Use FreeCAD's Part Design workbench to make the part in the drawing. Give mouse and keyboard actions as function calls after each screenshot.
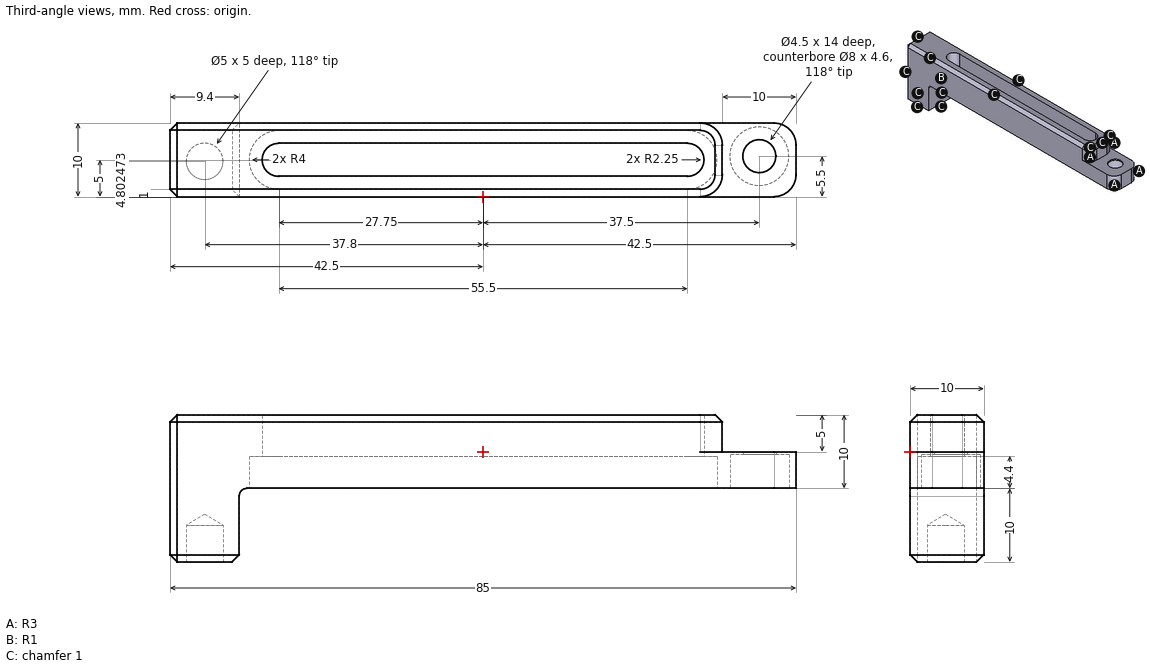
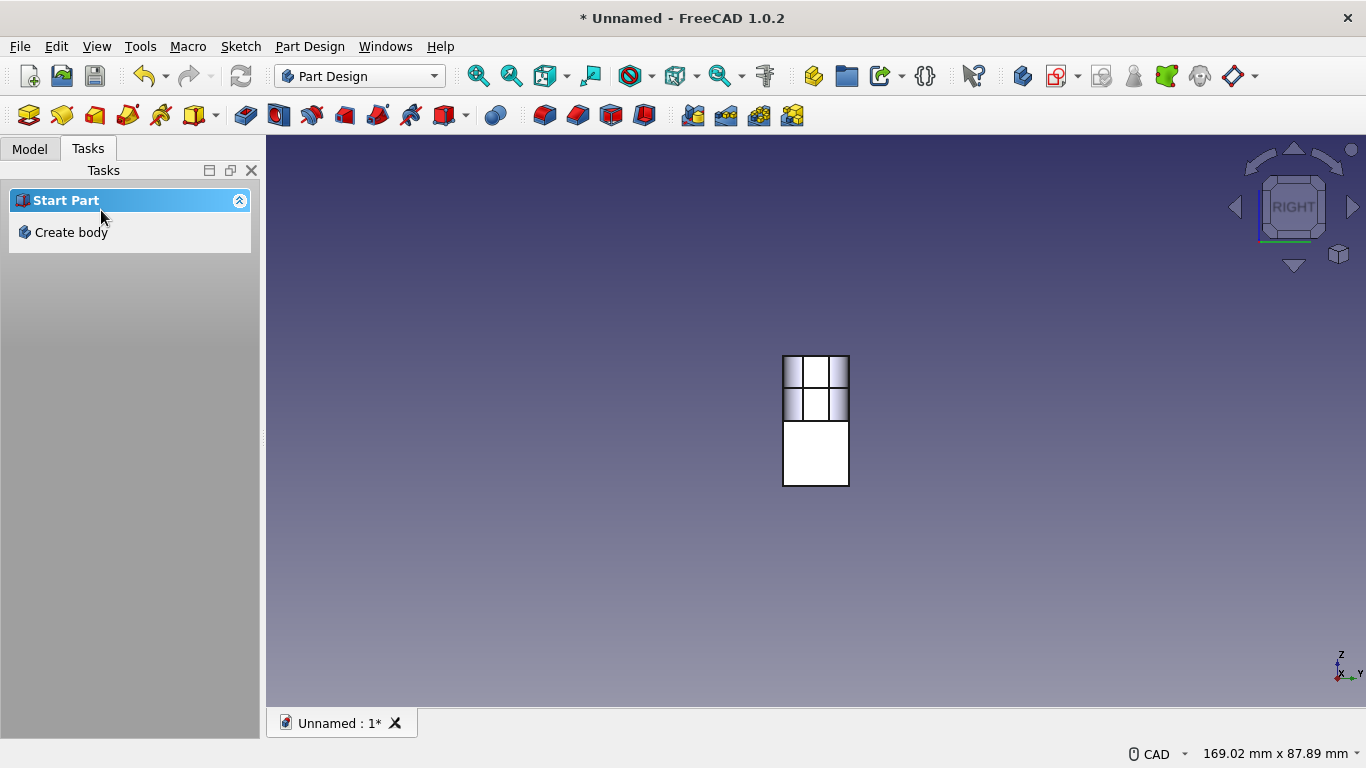
key(5)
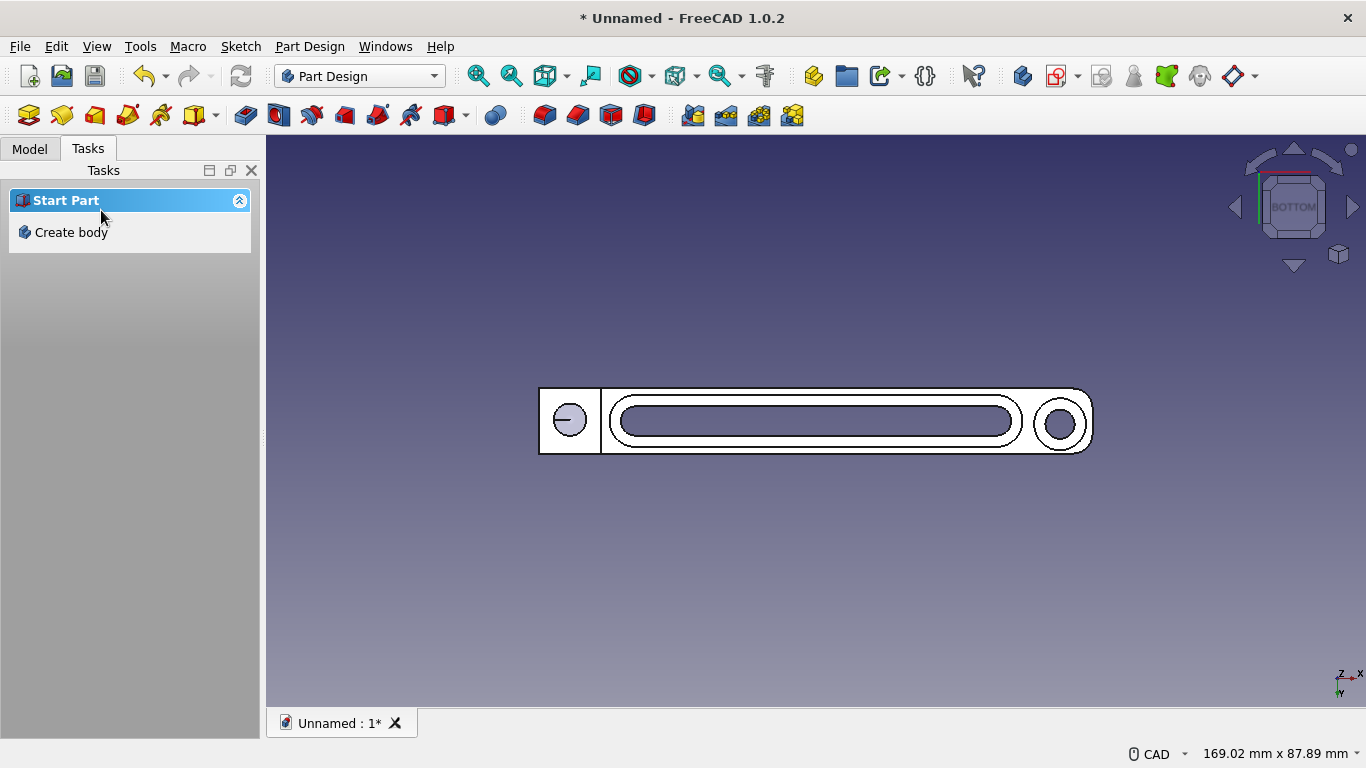
key(4)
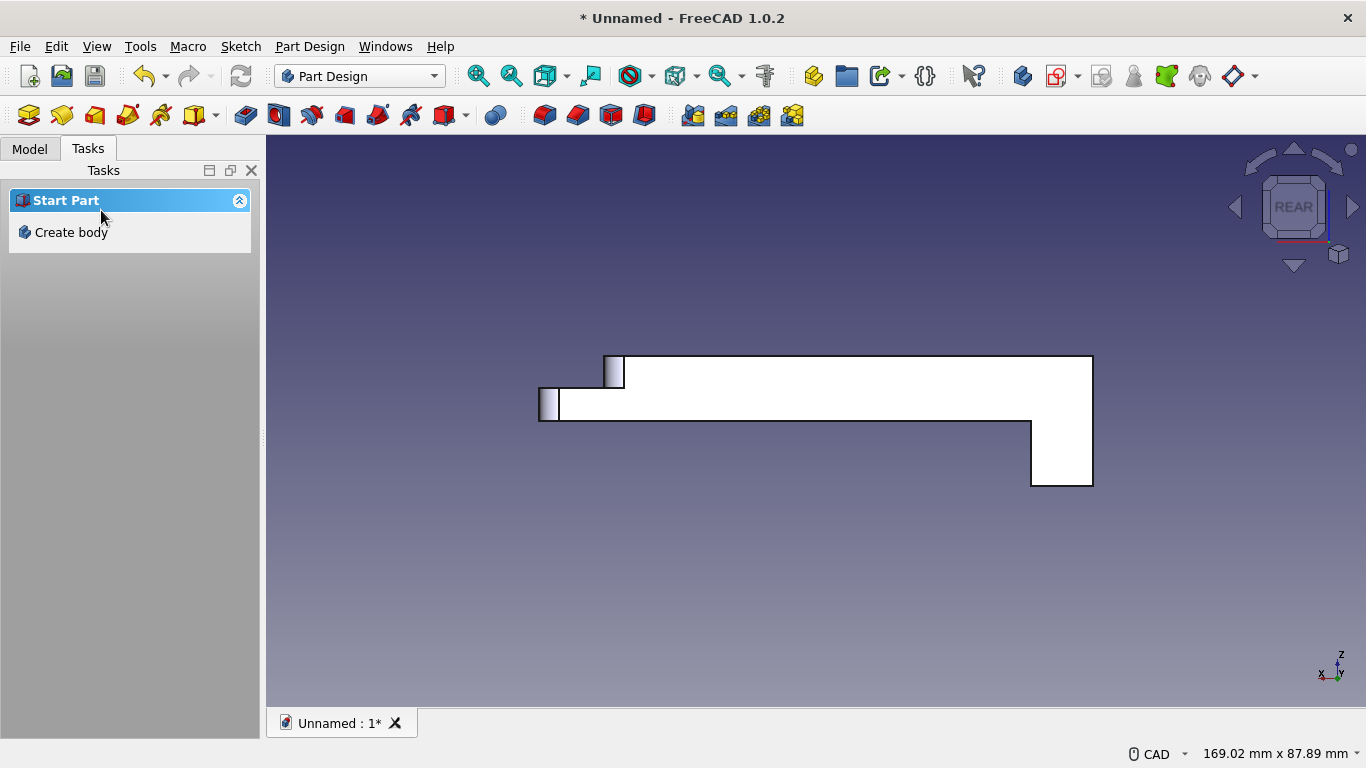
key(6)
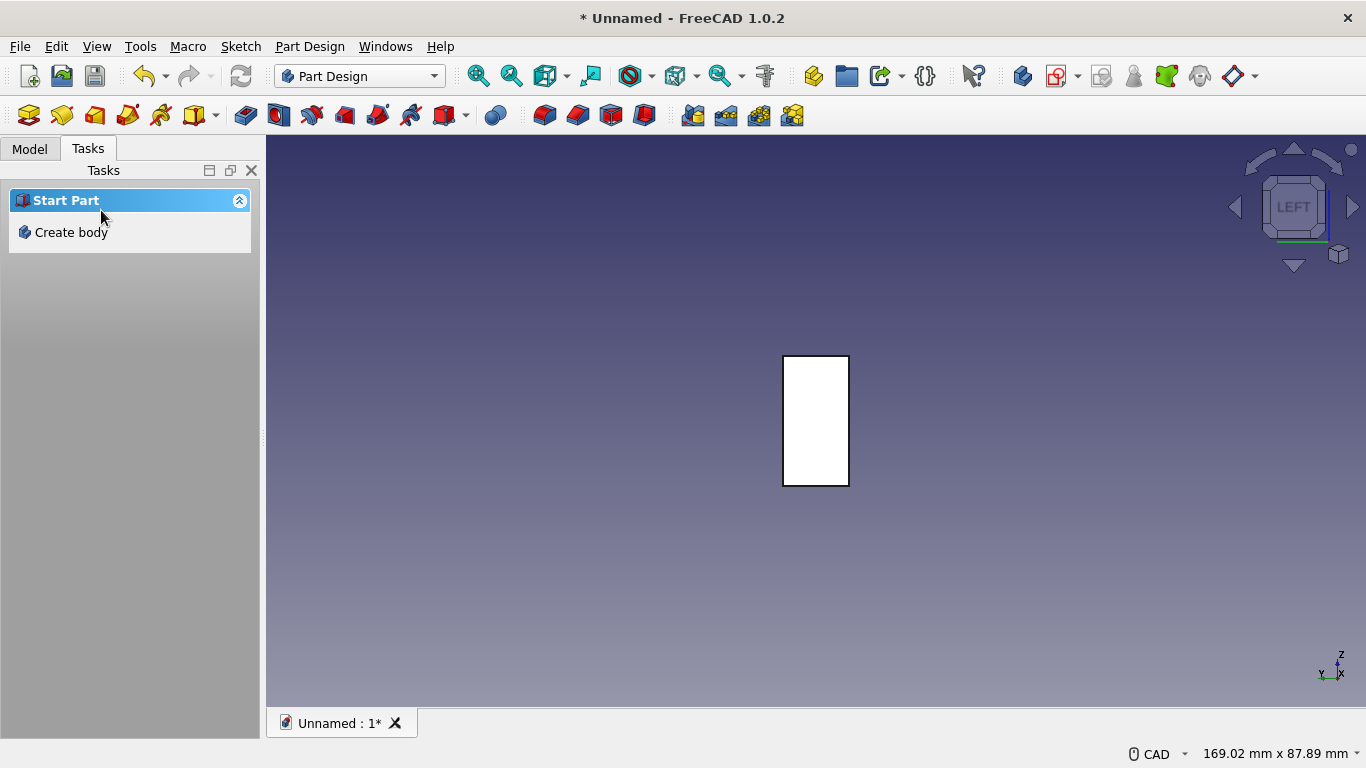
click(479, 76)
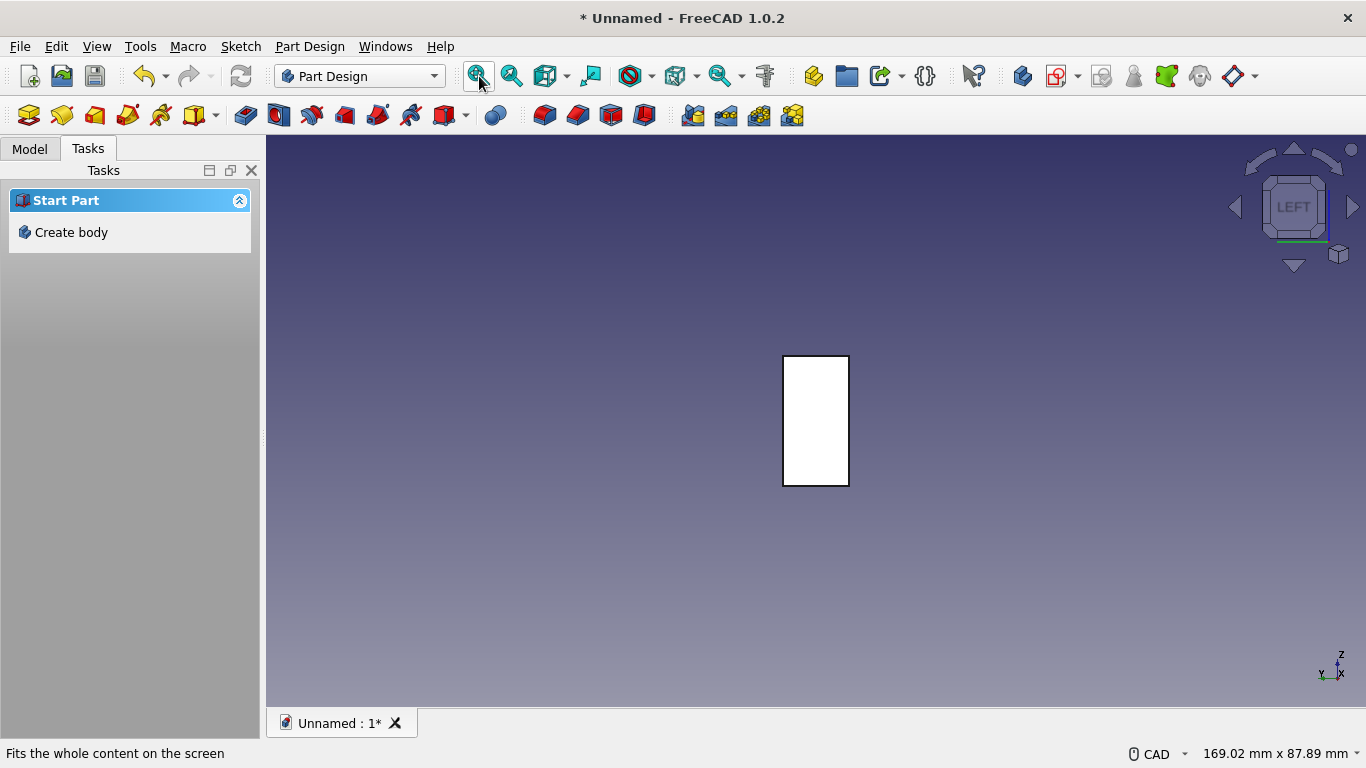
key(v)
key(3)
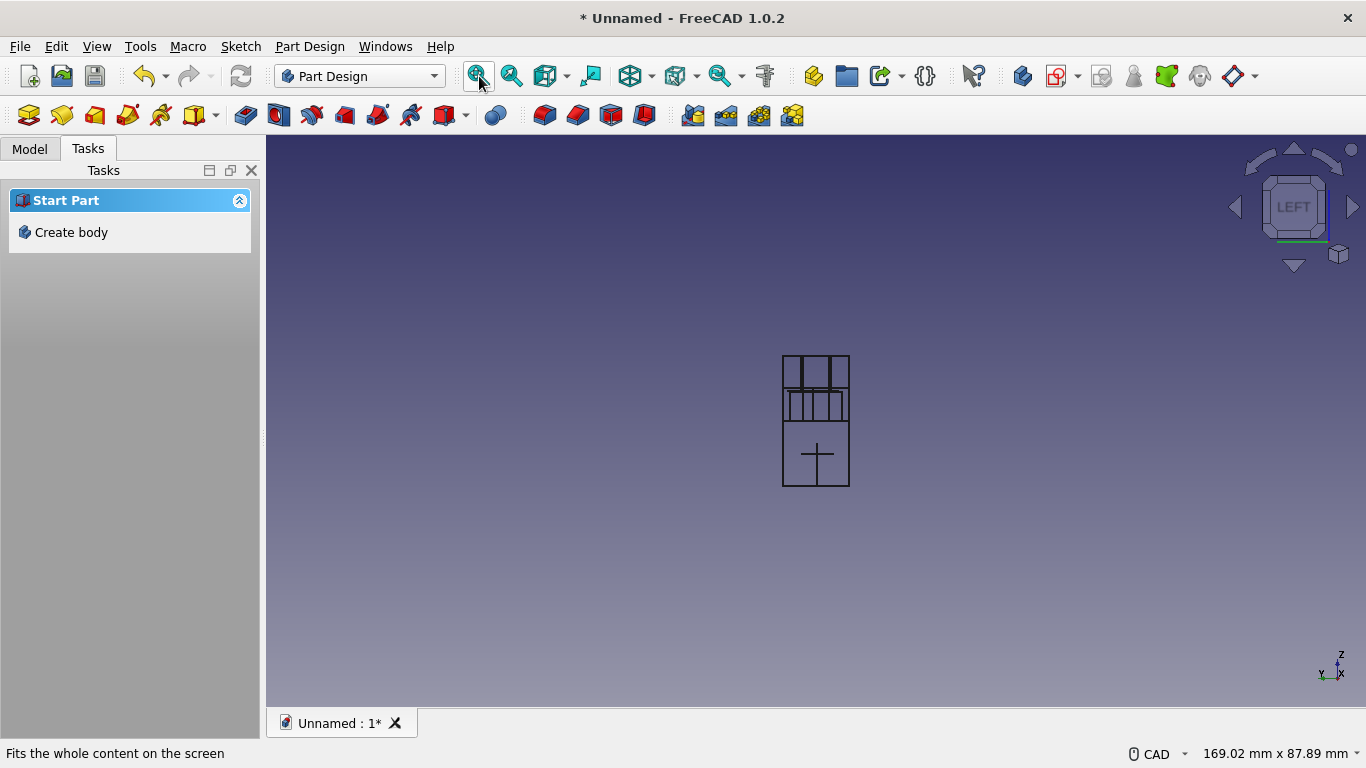
key(0)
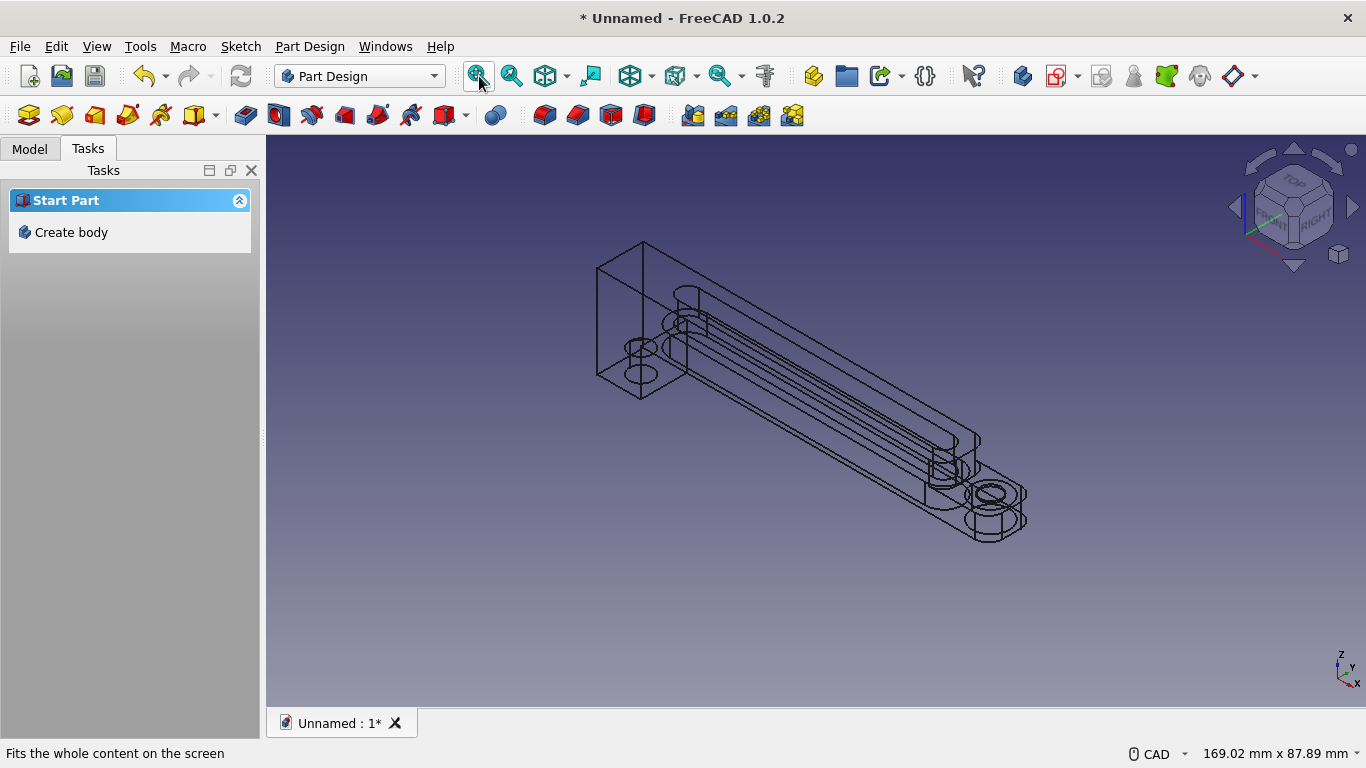
click(659, 335)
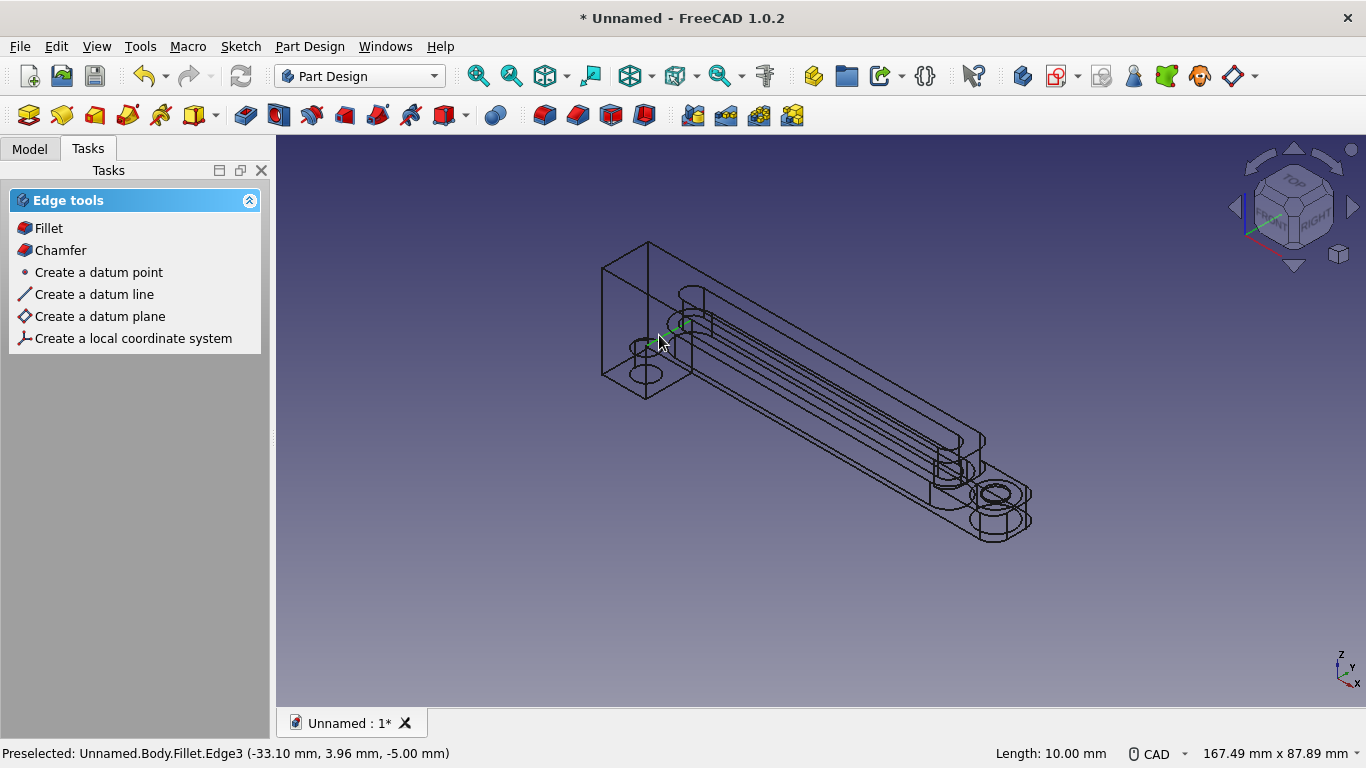
key(v)
key(1)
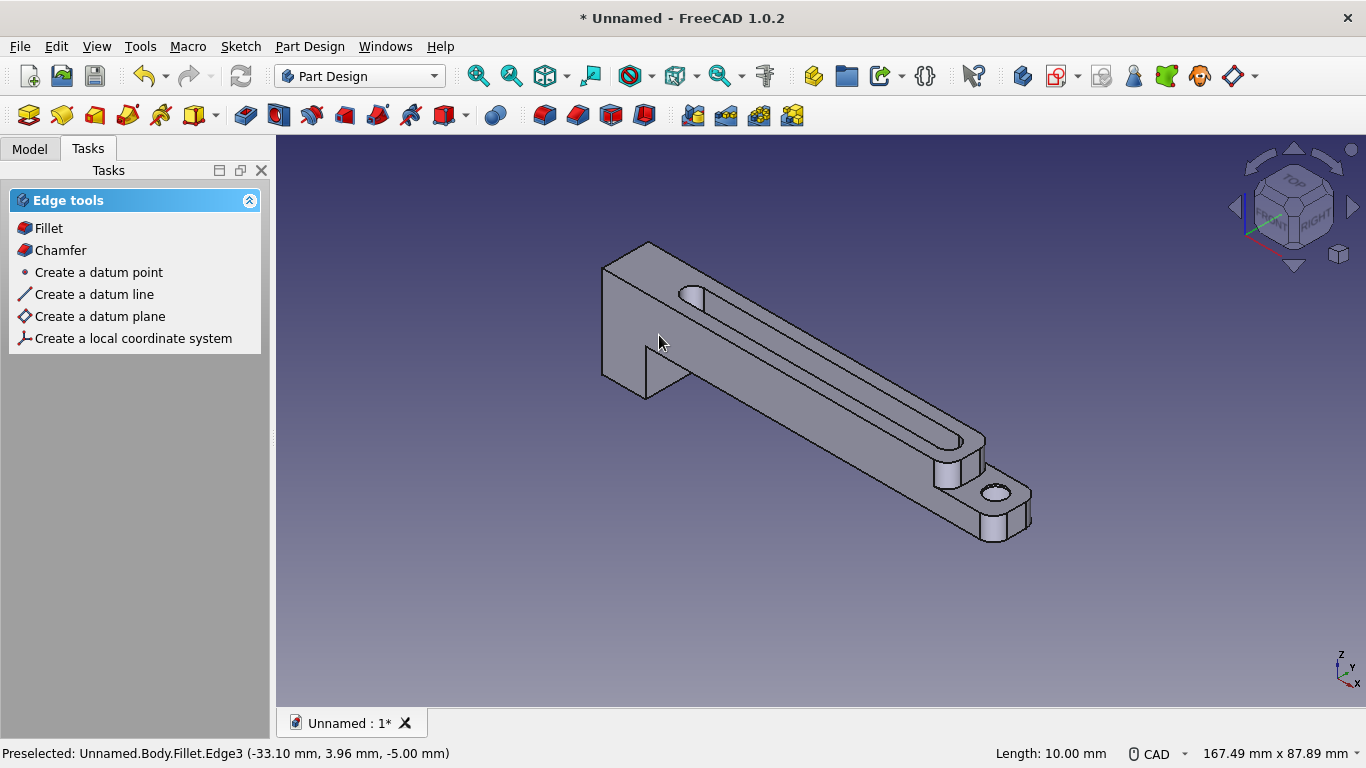
click(545, 116)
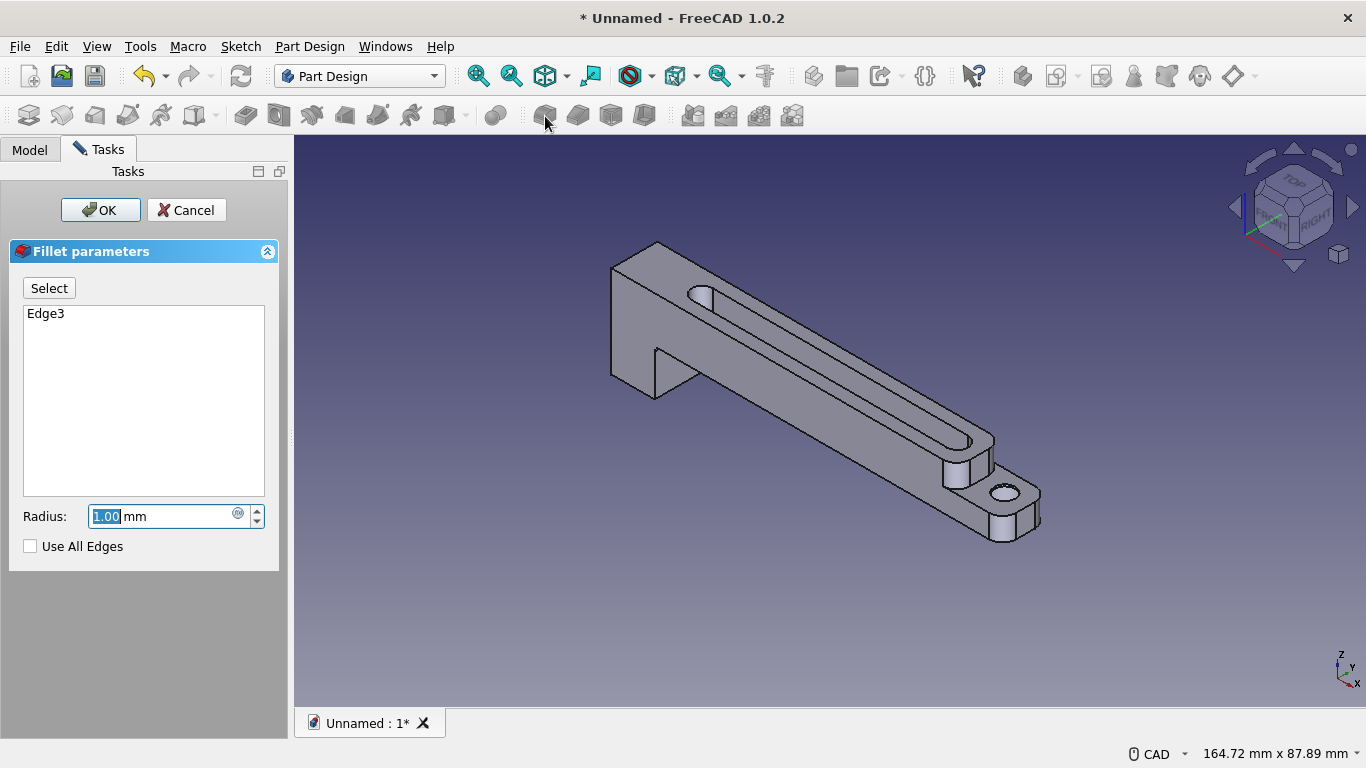
text(1)
key(Tab)